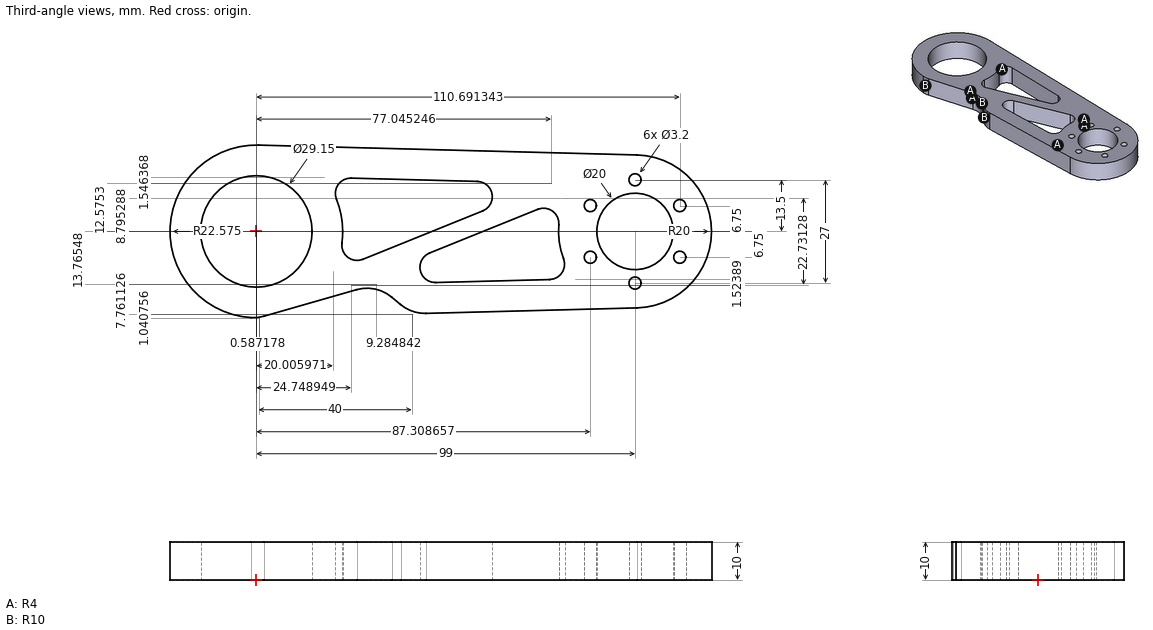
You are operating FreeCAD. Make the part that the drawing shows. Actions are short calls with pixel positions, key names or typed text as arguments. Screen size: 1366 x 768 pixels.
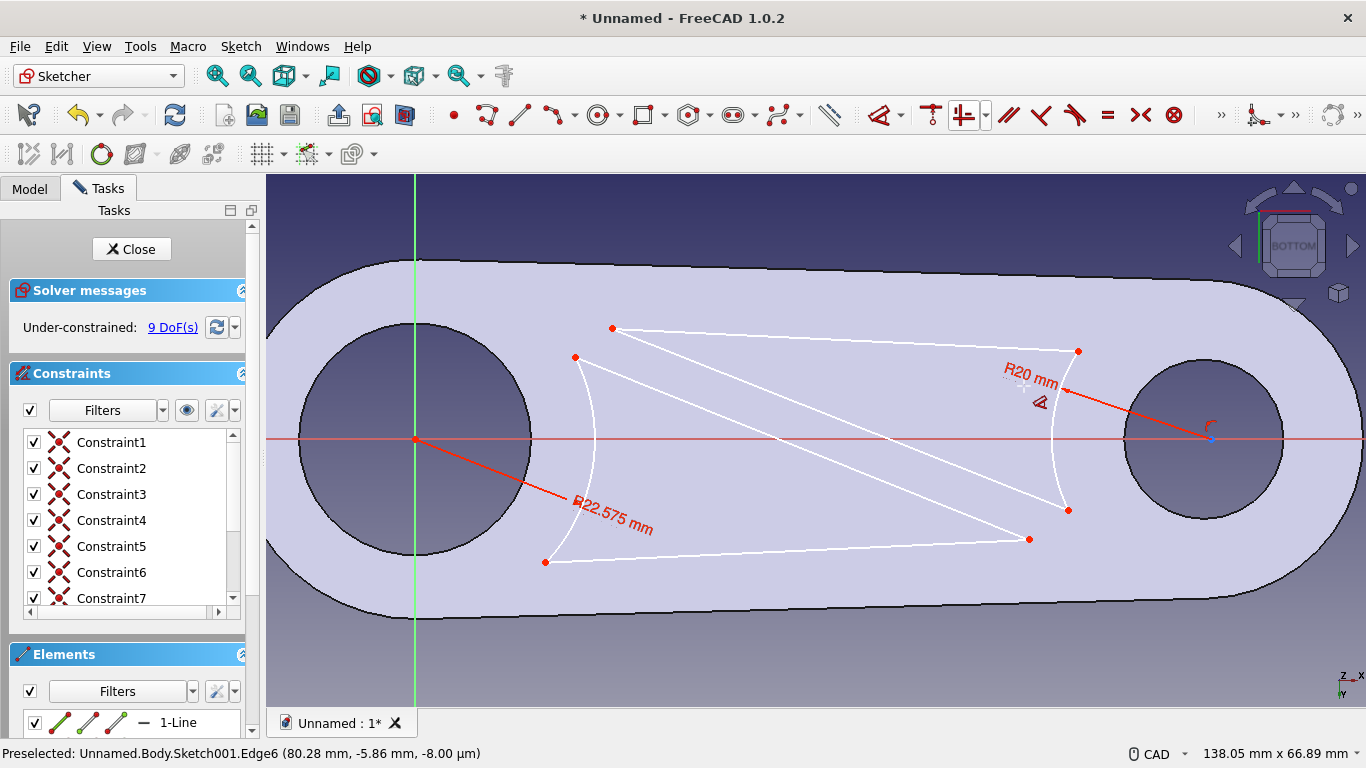
scroll(451, 443, down, 1)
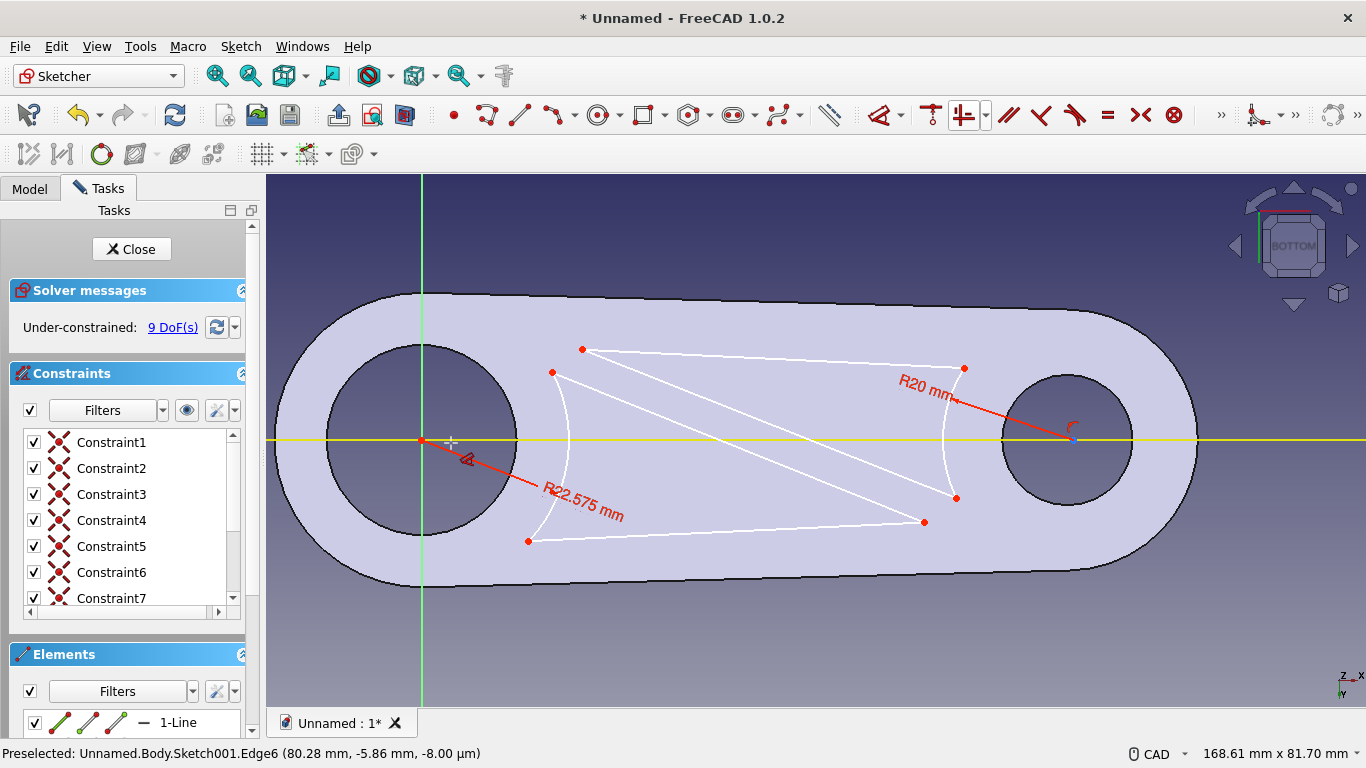
click(1074, 440)
click(598, 406)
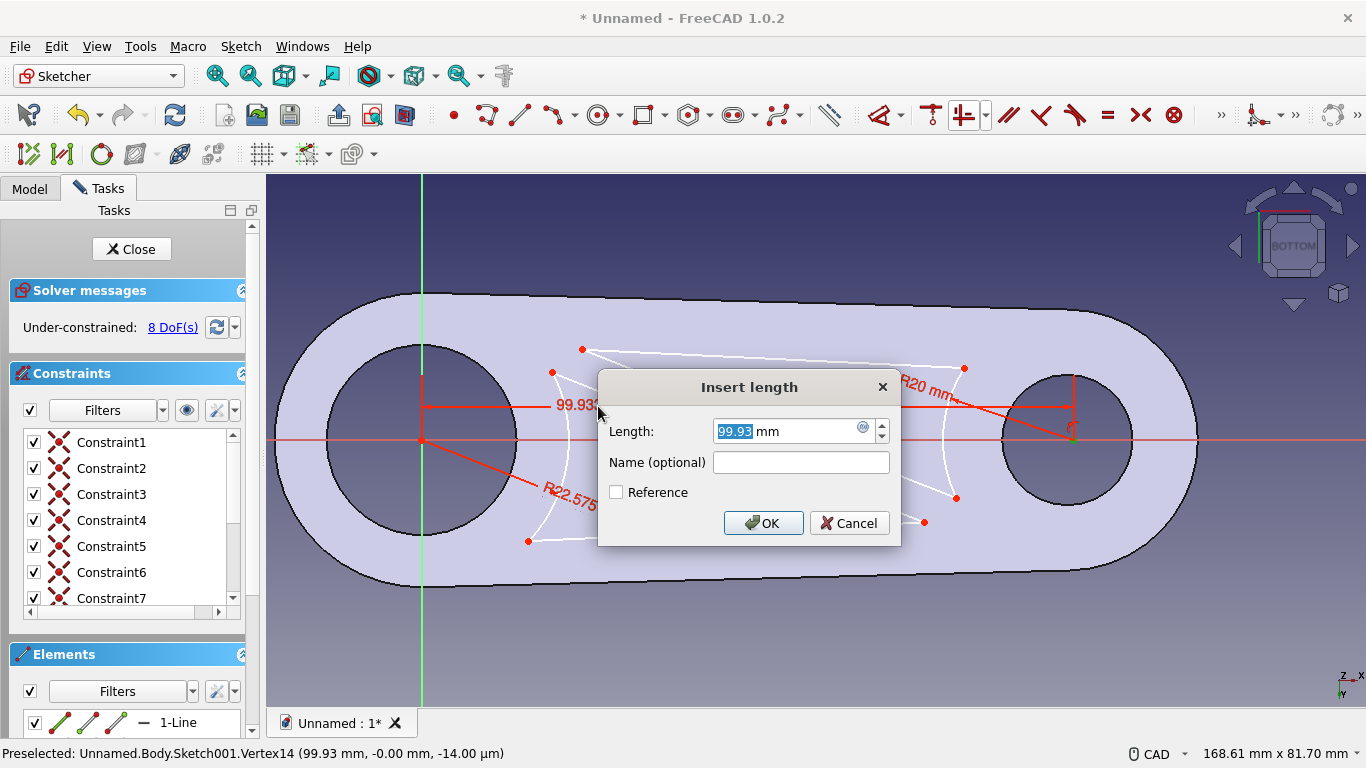
text(99)
key(Return)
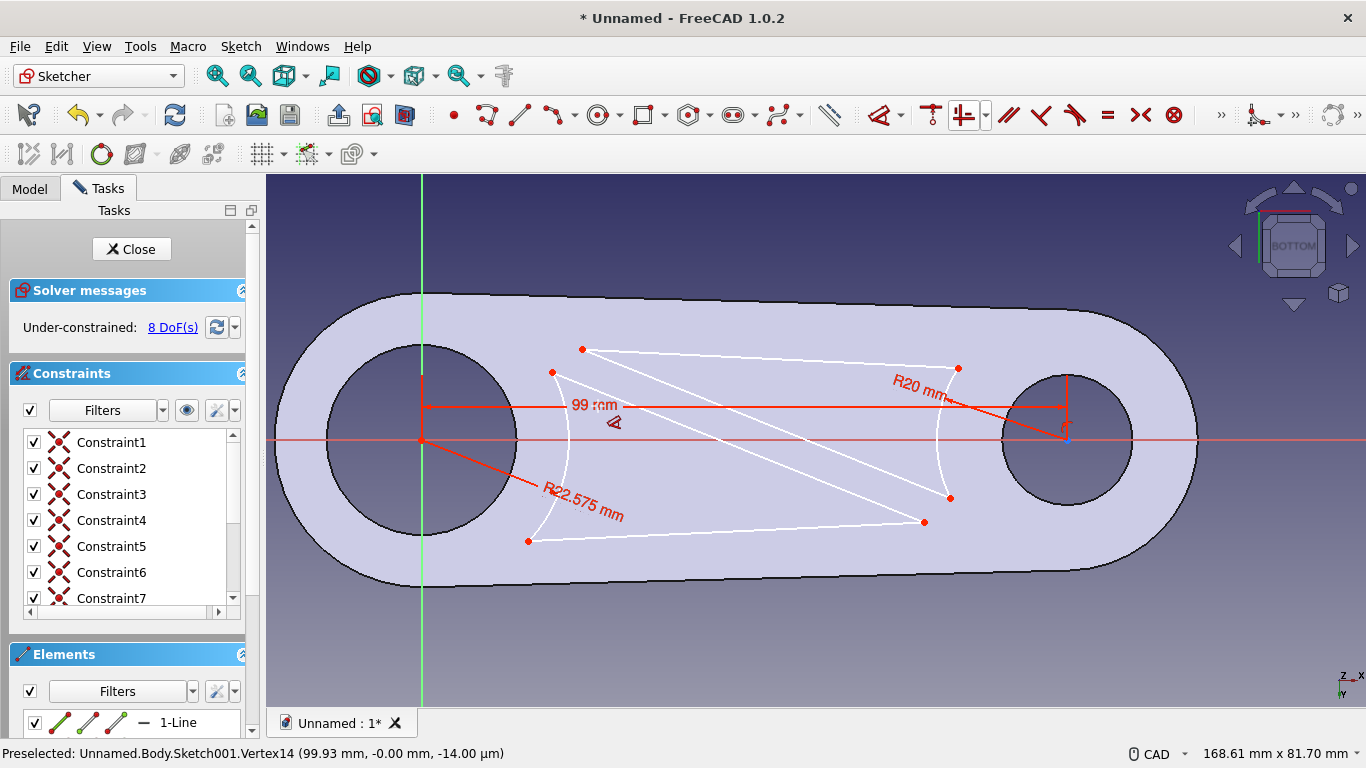
click(924, 523)
click(388, 481)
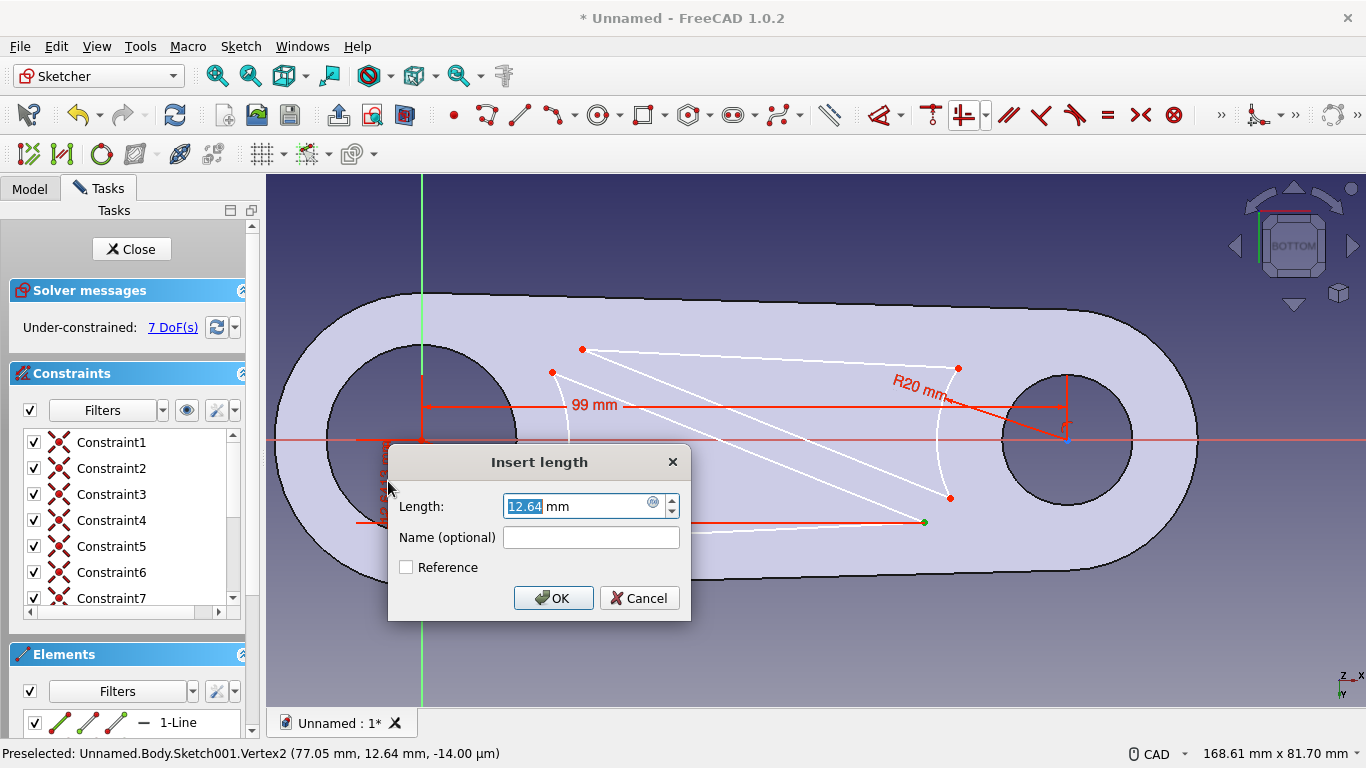
text(12.5753)
key(Return)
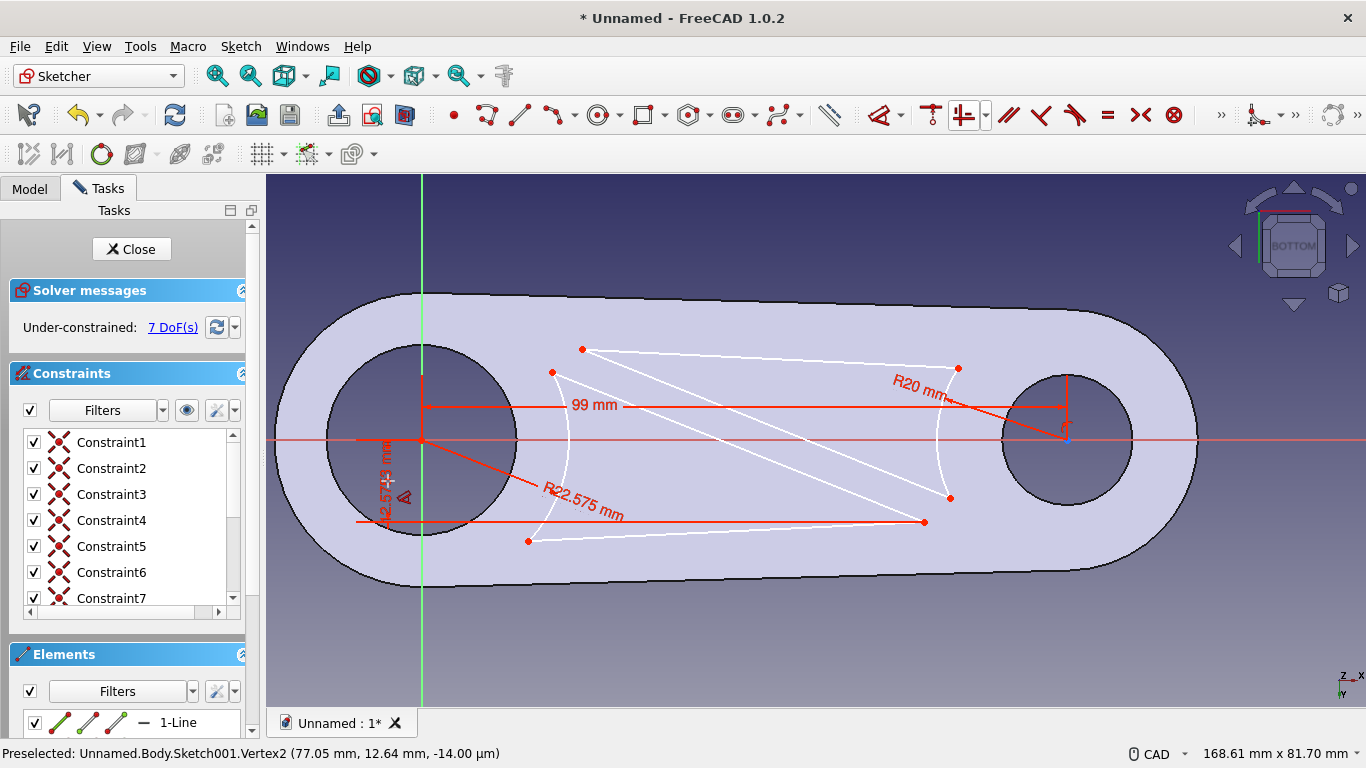
scroll(696, 355, up, 7)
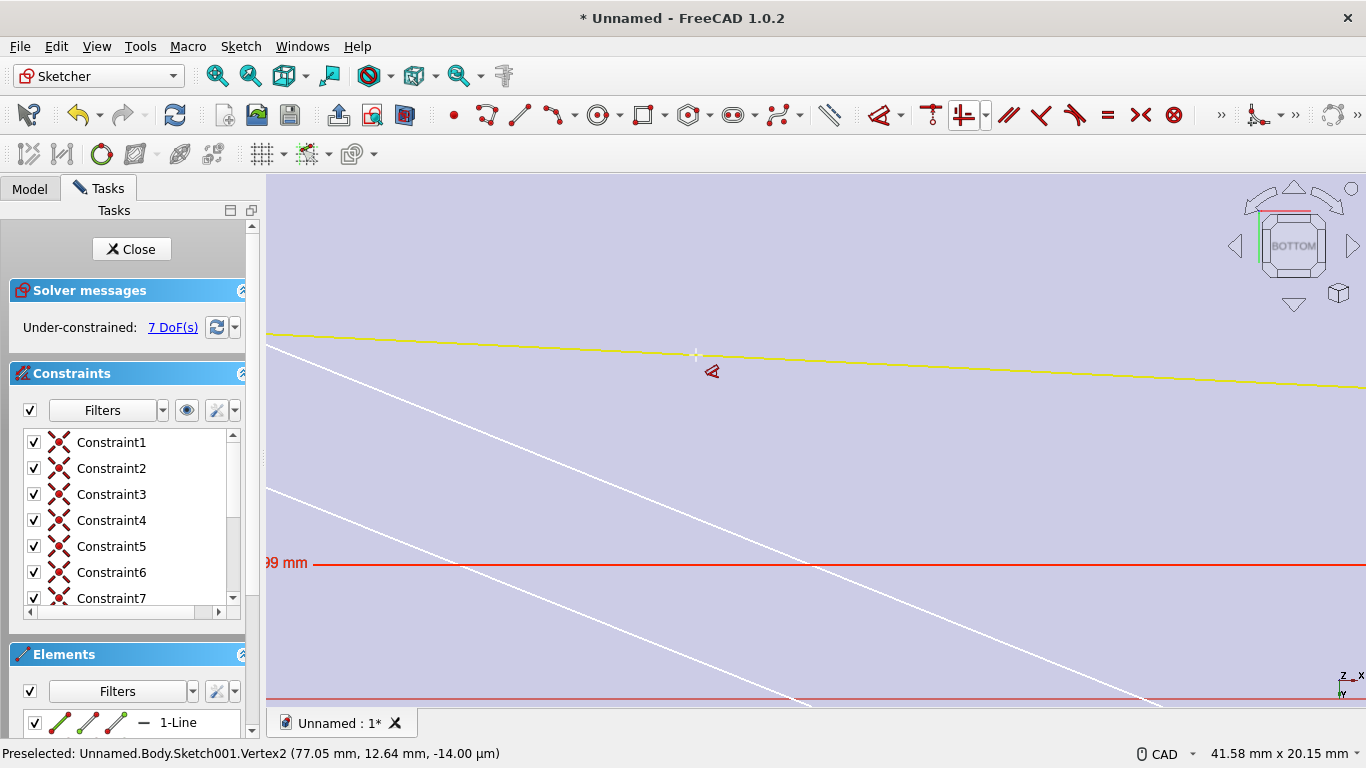
click(693, 355)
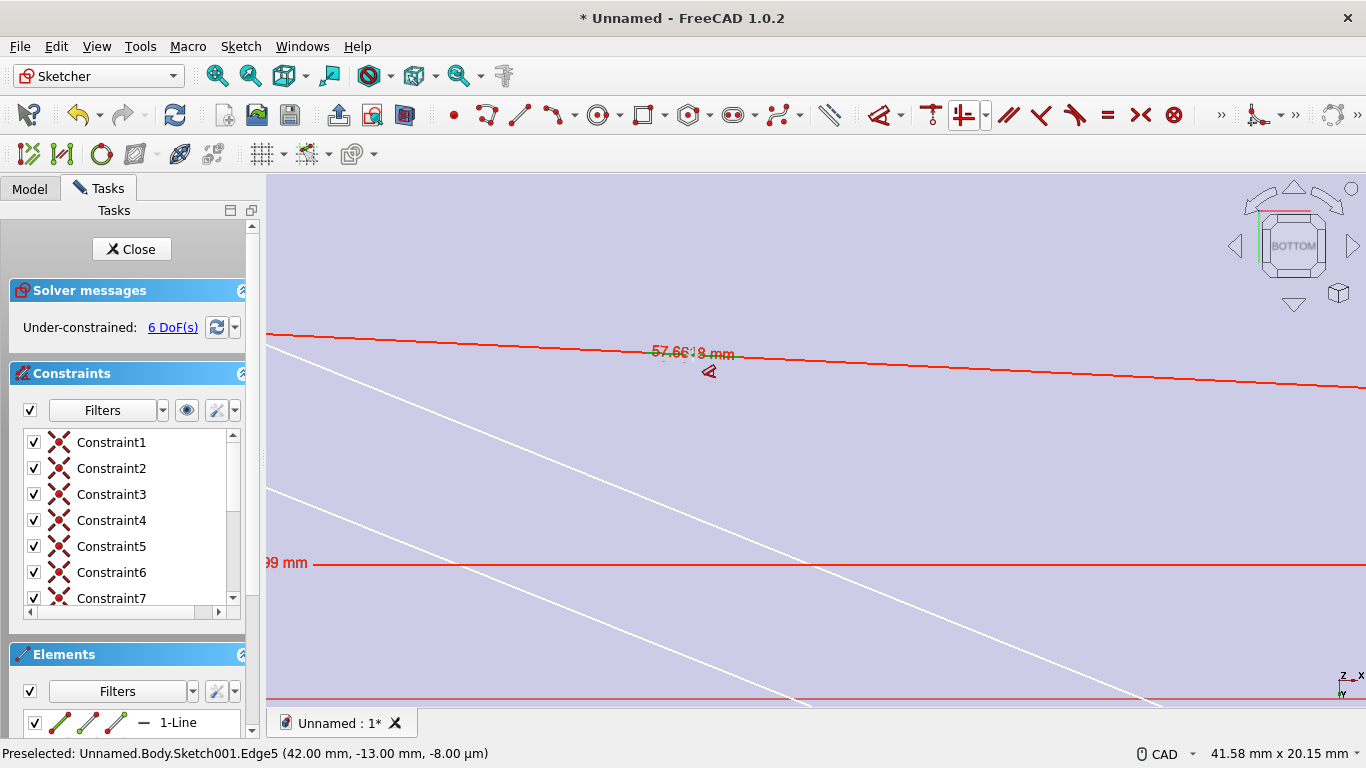
key(Escape)
key(Escape)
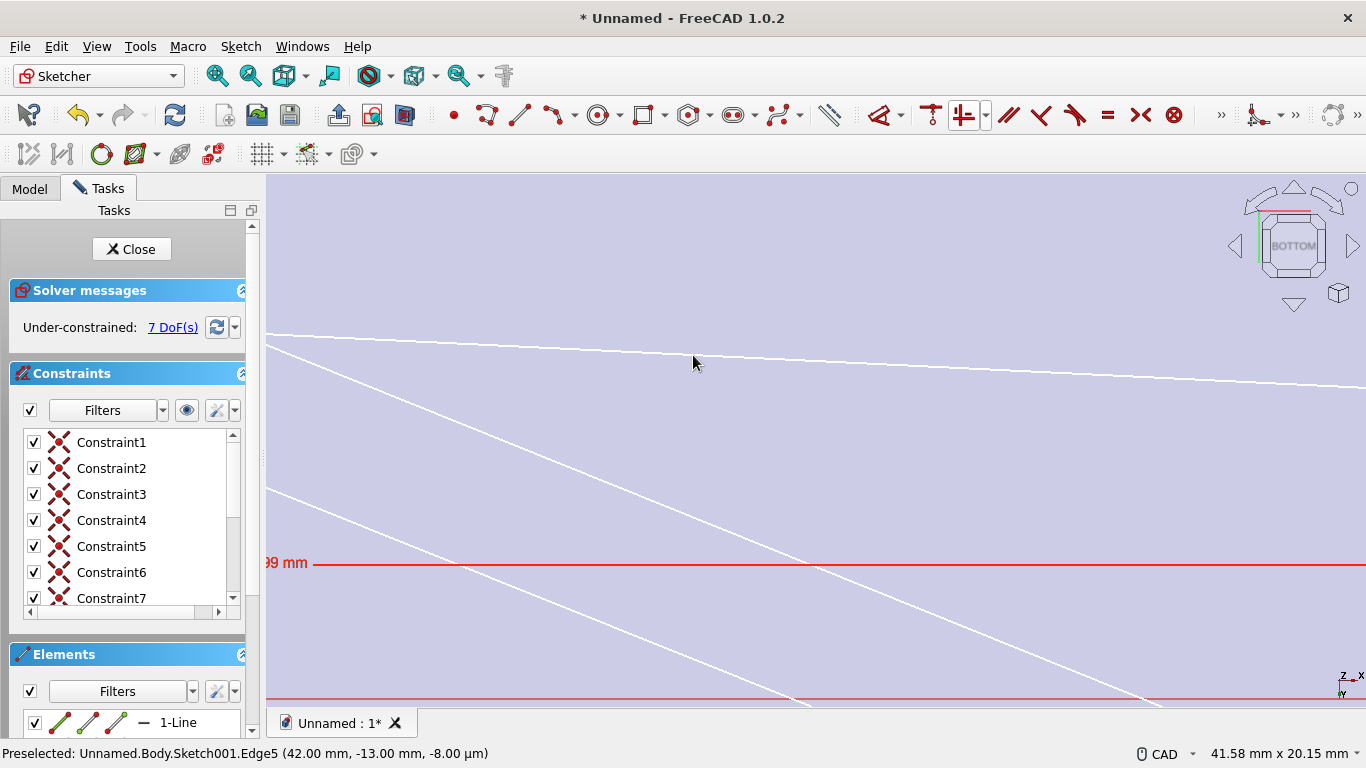
click(693, 355)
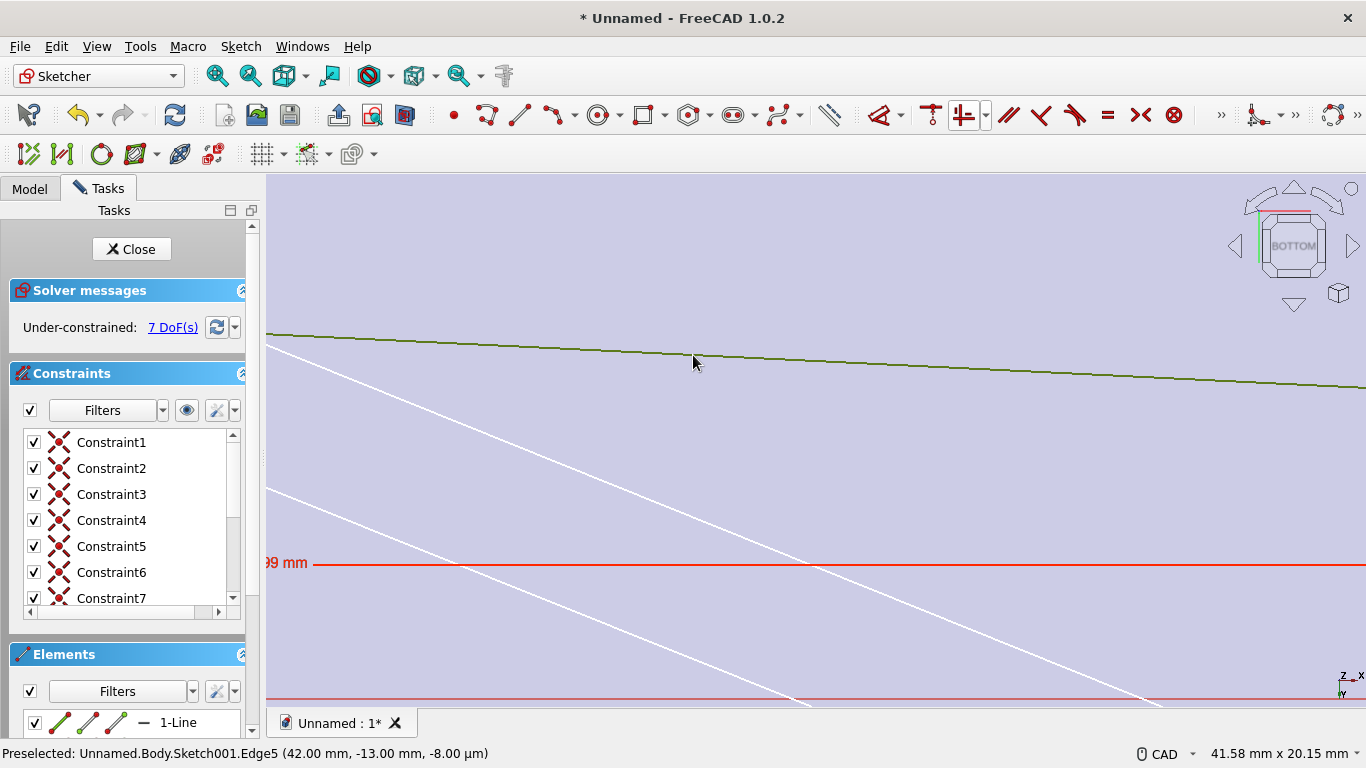
key(i)